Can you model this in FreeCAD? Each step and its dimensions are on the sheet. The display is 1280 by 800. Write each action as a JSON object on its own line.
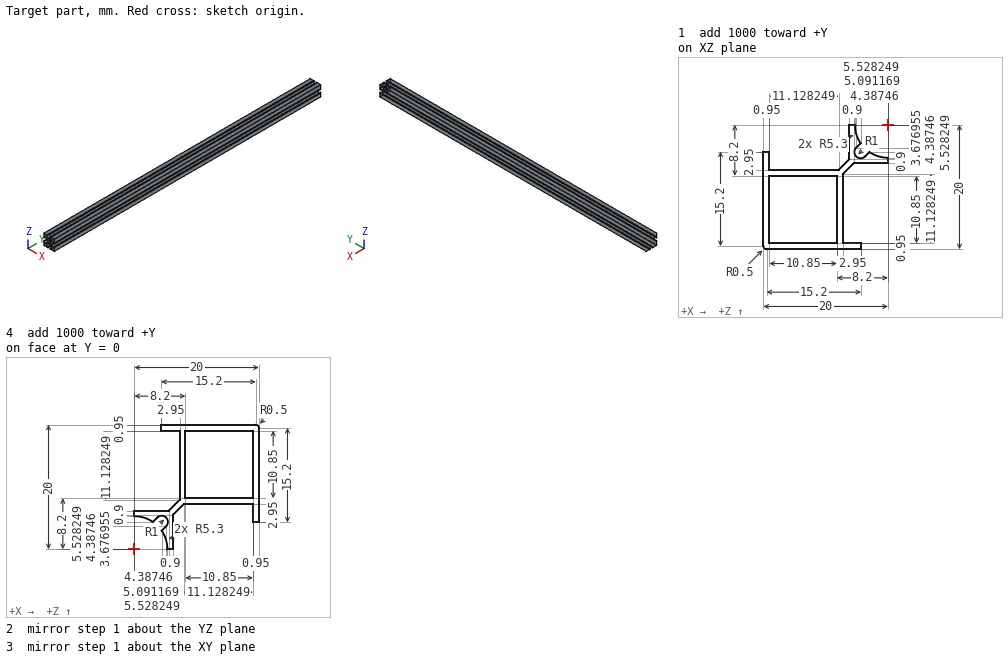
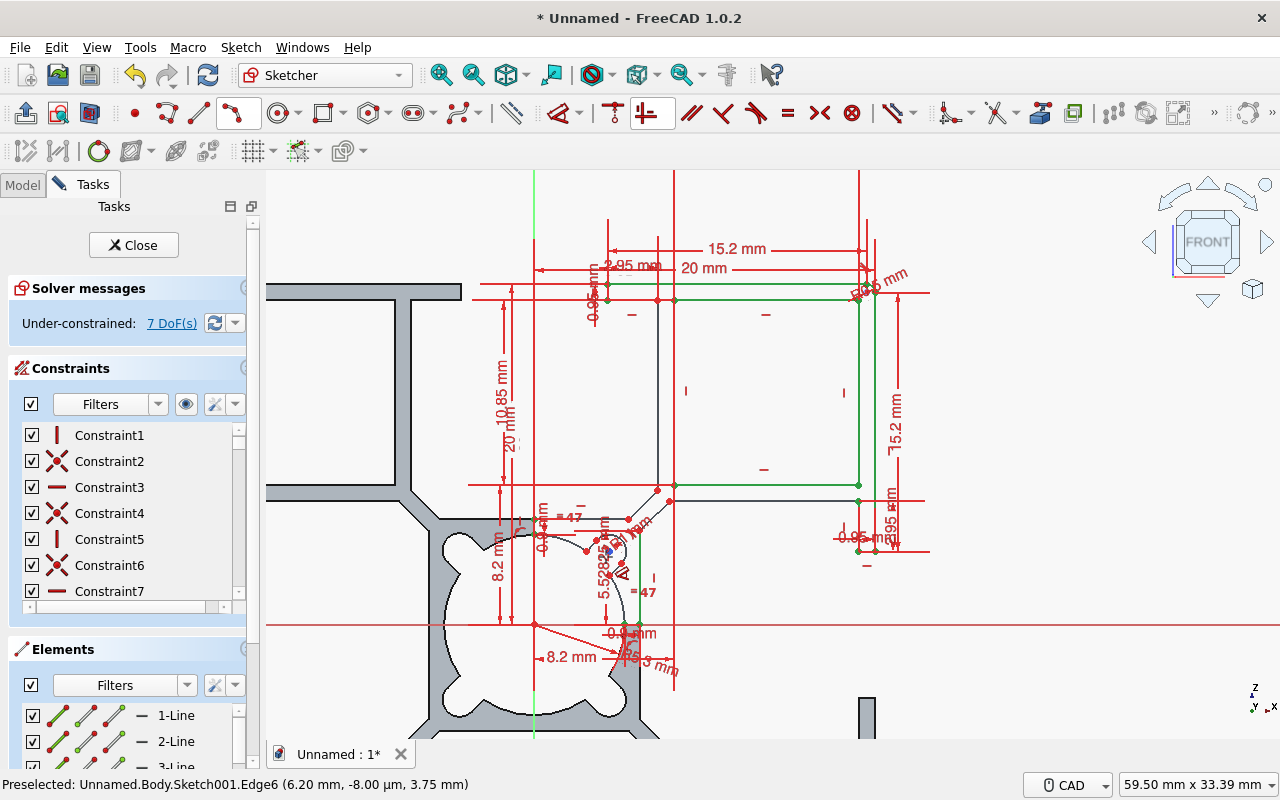
{"action": "left_click", "coordinate": [563, 519]}
{"action": "left_click", "coordinate": [582, 485]}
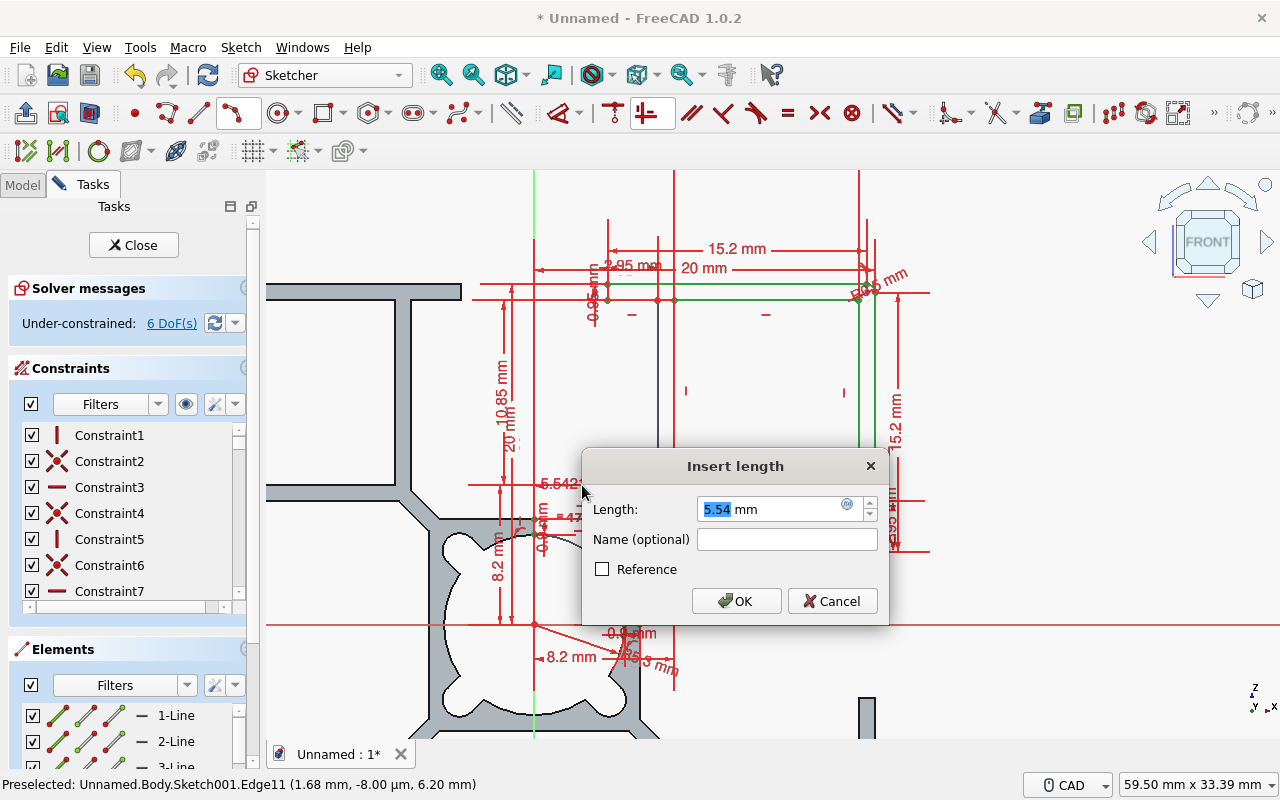
{"action": "type", "text": "5.528249"}
{"action": "key", "text": "Return"}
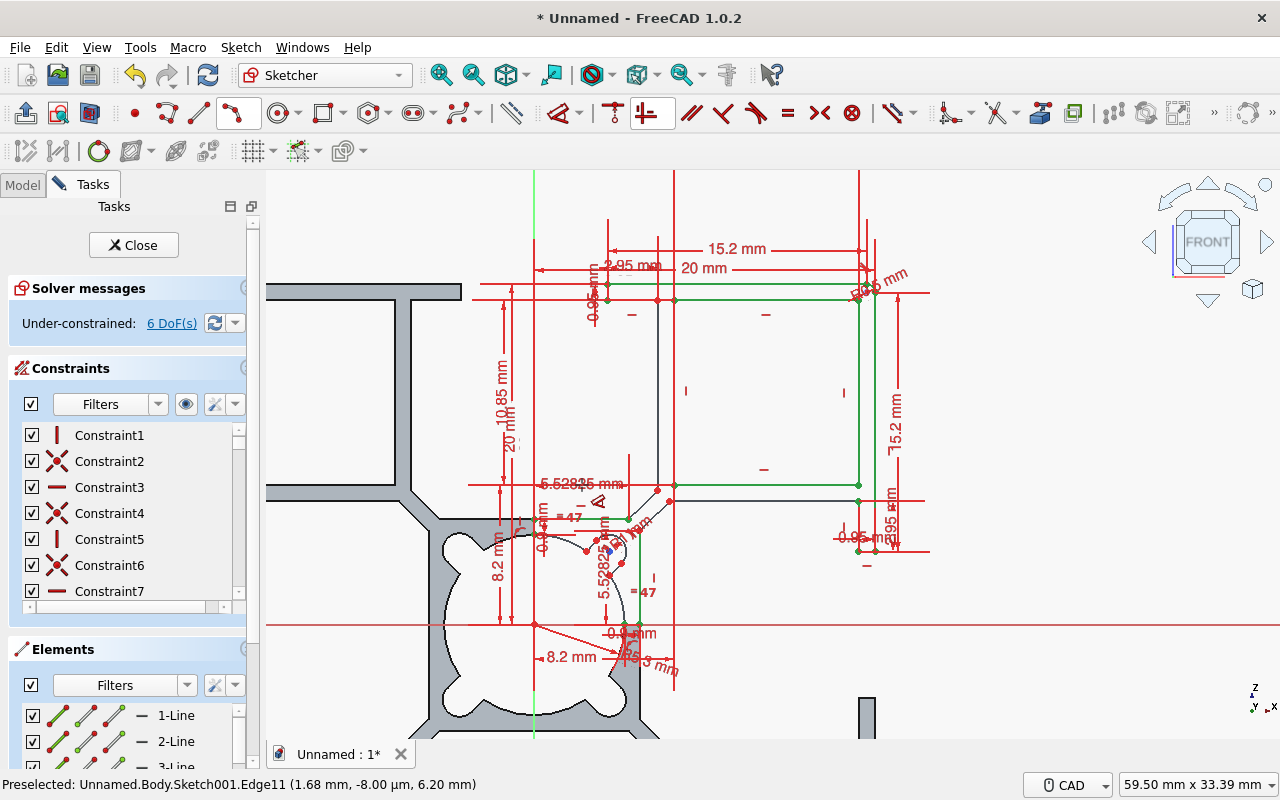
{"action": "left_click", "coordinate": [610, 576]}
{"action": "left_click", "coordinate": [572, 683]}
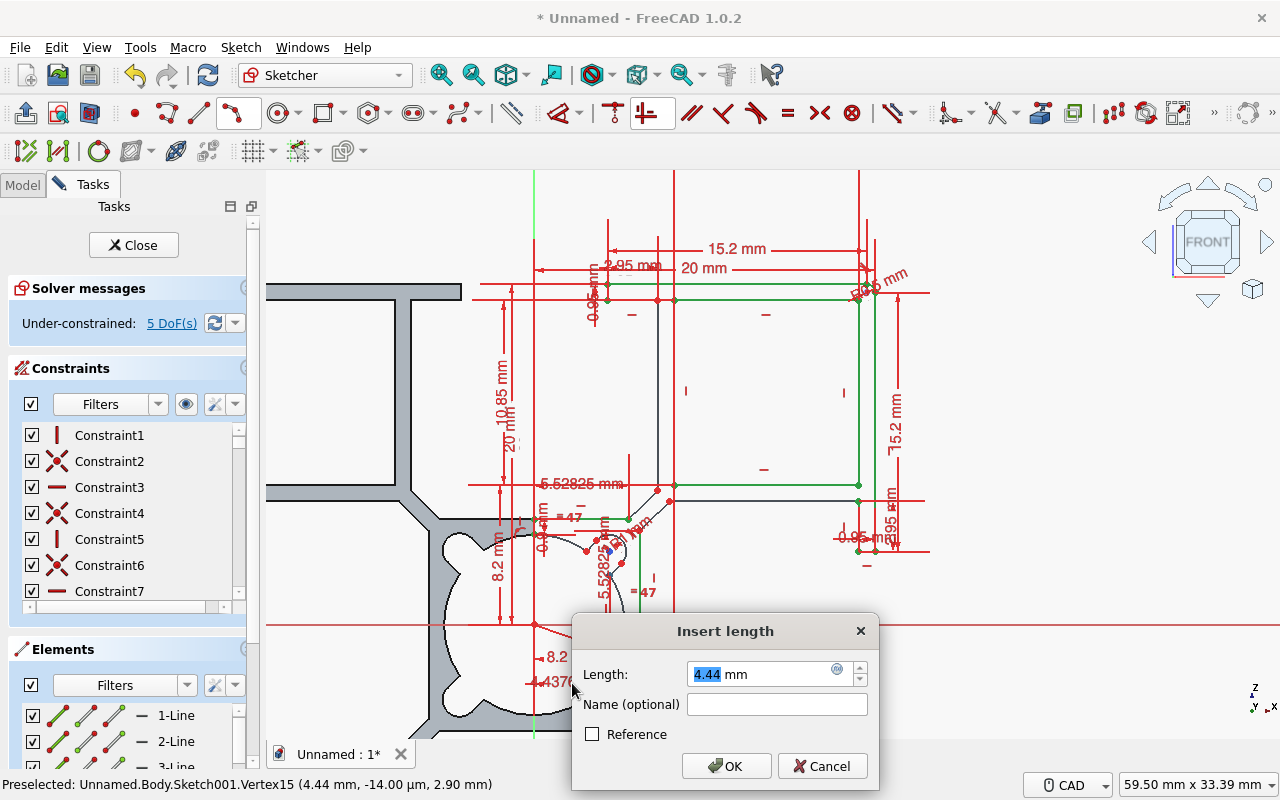
{"action": "type", "text": "4.38746"}
{"action": "key", "text": "Return"}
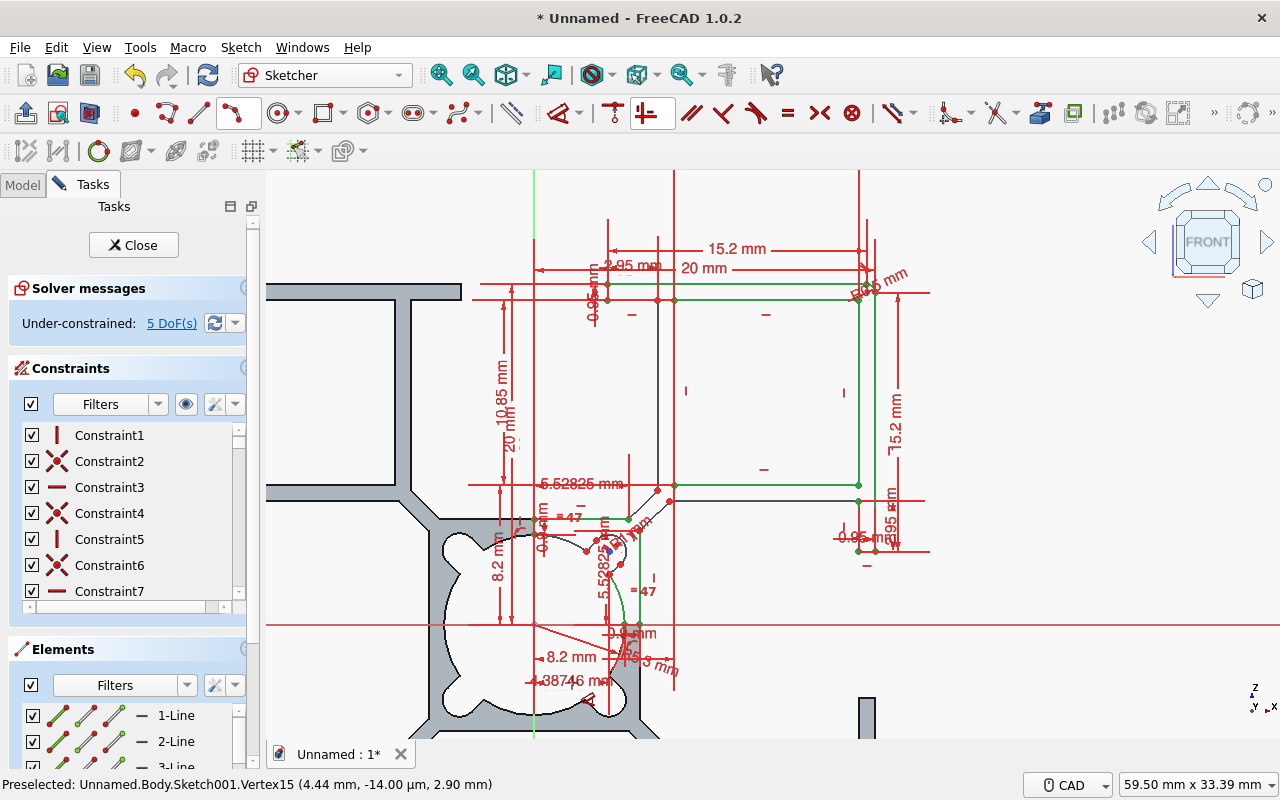
{"action": "left_click", "coordinate": [587, 552]}
{"action": "left_click", "coordinate": [500, 588]}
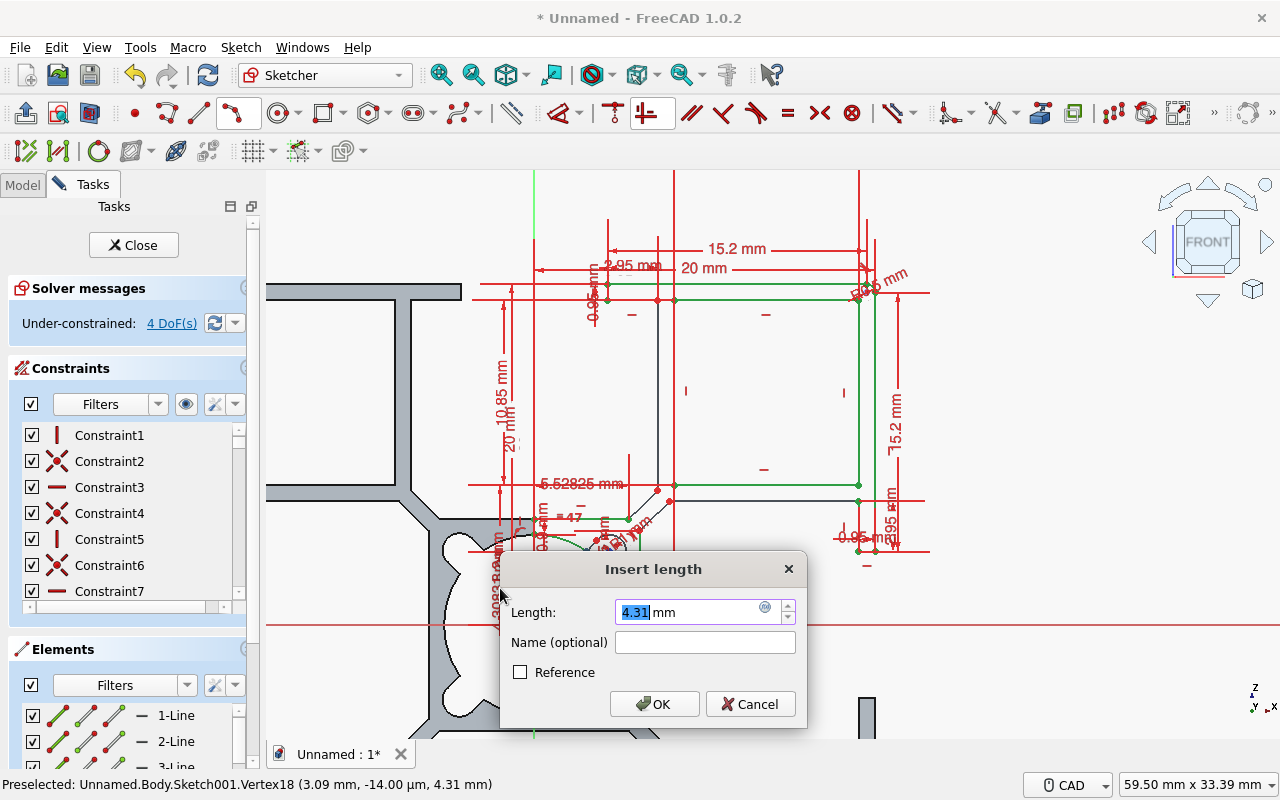
{"action": "type", "text": "4.38746"}
{"action": "key", "text": "Return"}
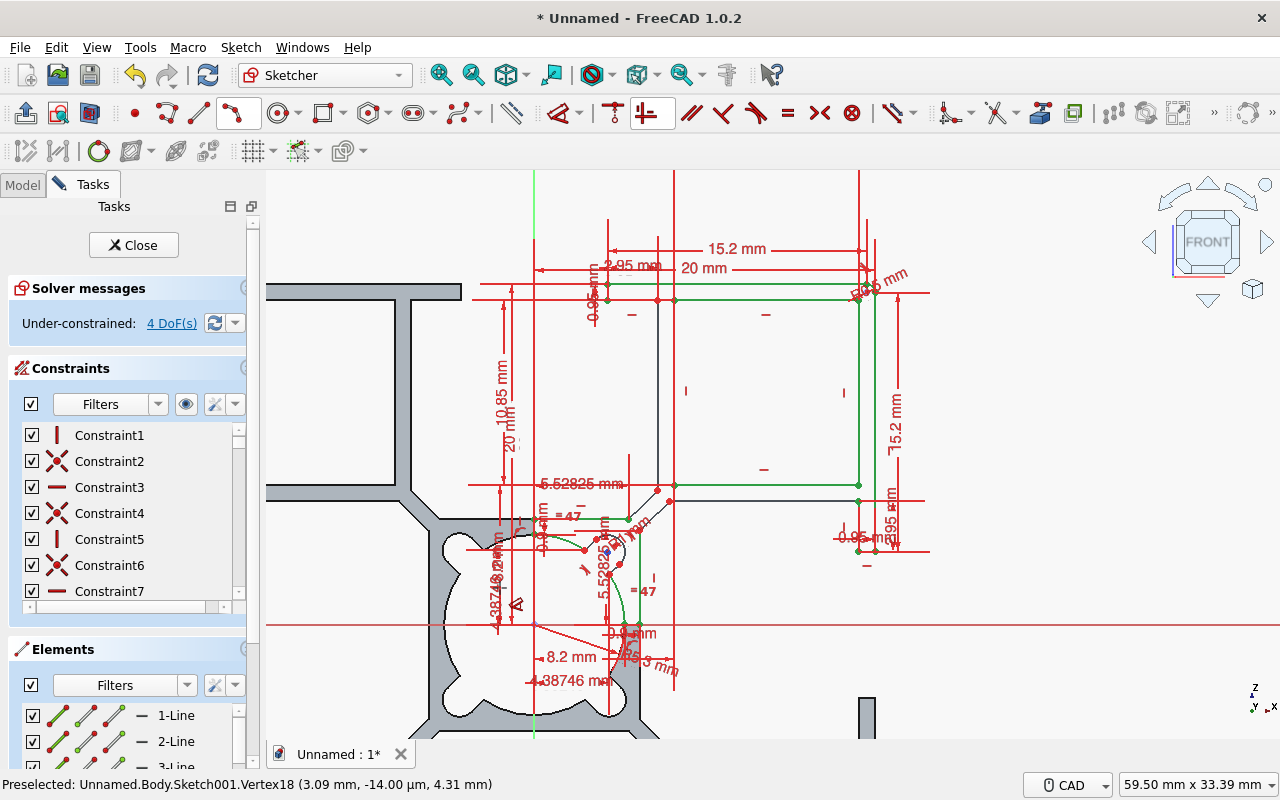
{"action": "left_click", "coordinate": [802, 501]}
{"action": "left_click", "coordinate": [764, 535]}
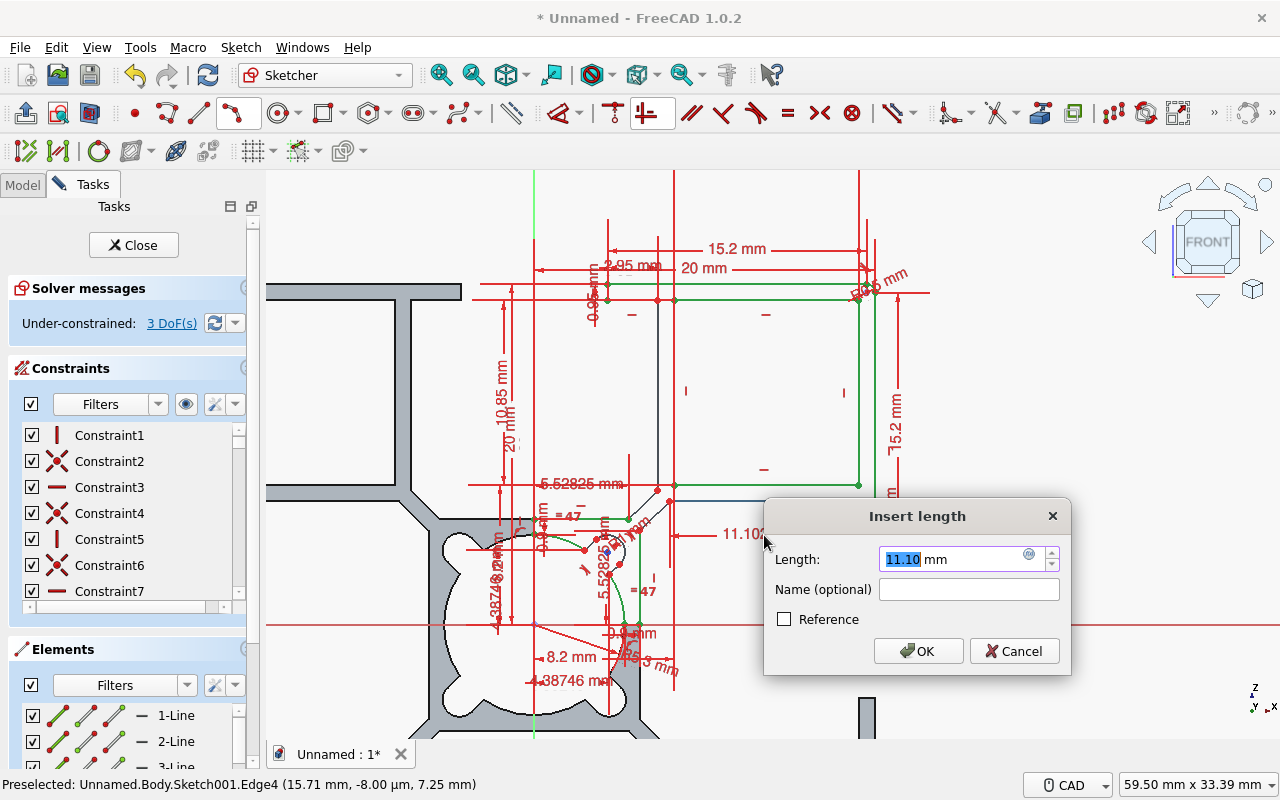
{"action": "type", "text": "11.128249"}
{"action": "key", "text": "Return"}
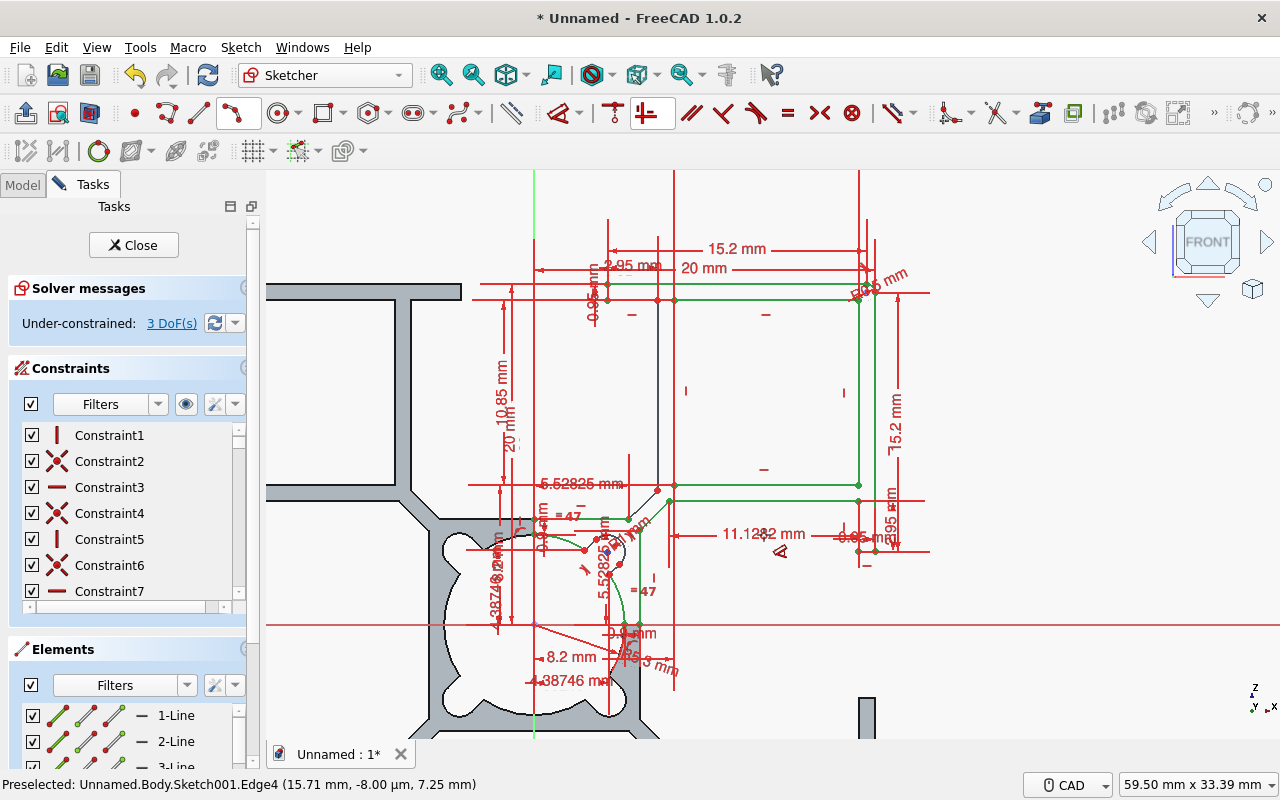
{"action": "left_click", "coordinate": [658, 434]}
{"action": "left_click", "coordinate": [624, 396]}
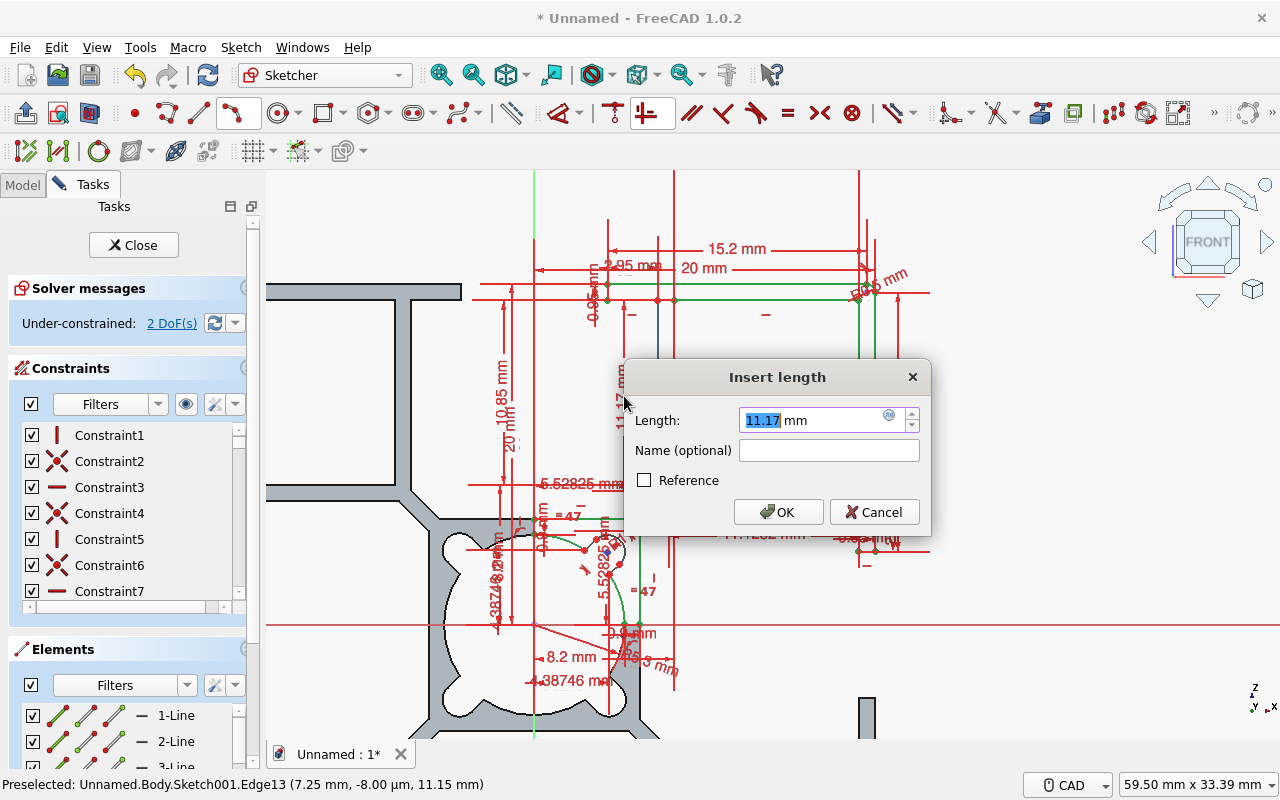
{"action": "type", "text": "11.128249"}
{"action": "key", "text": "Return"}